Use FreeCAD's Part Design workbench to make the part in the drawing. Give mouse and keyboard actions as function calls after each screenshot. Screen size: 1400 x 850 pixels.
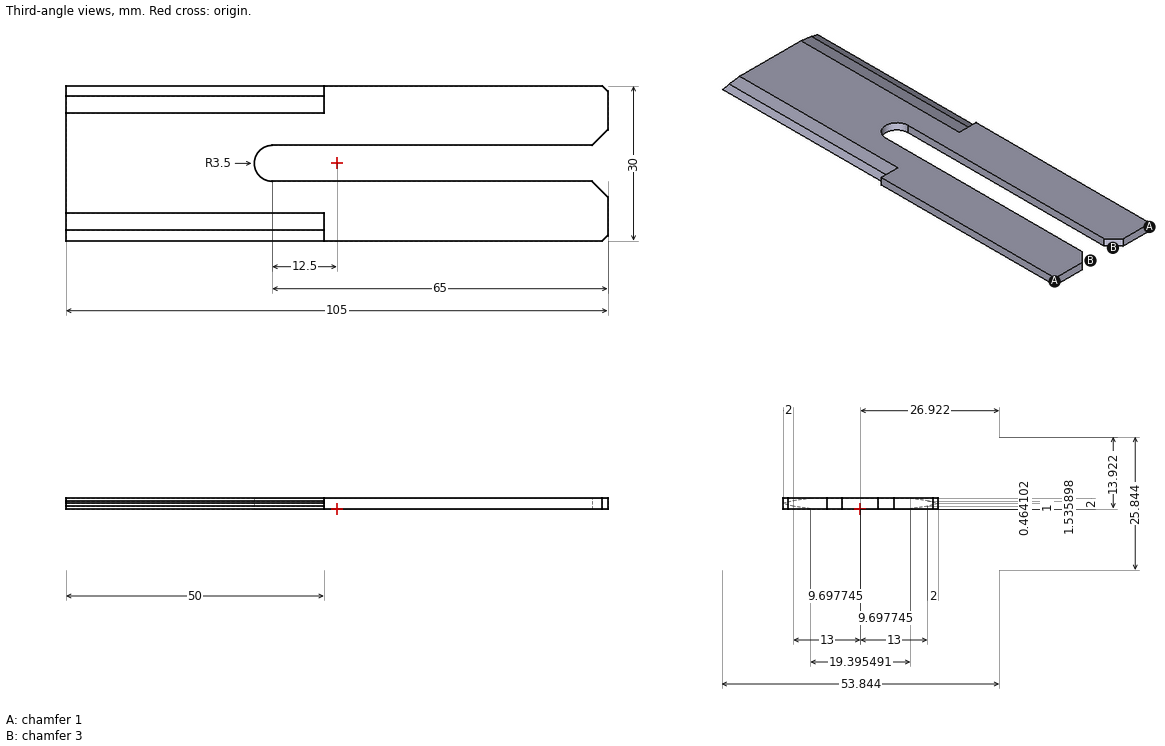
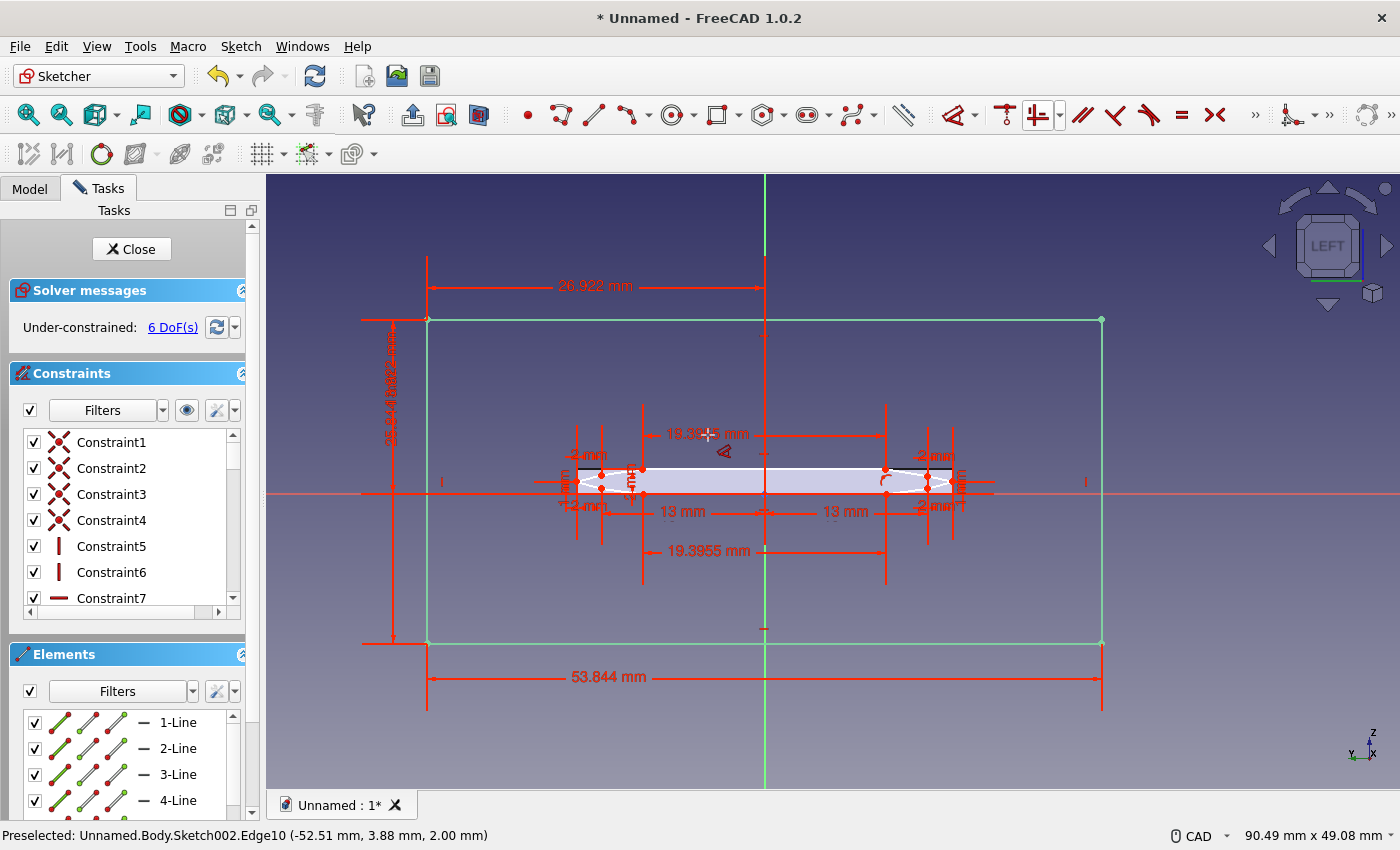
click(886, 494)
click(825, 552)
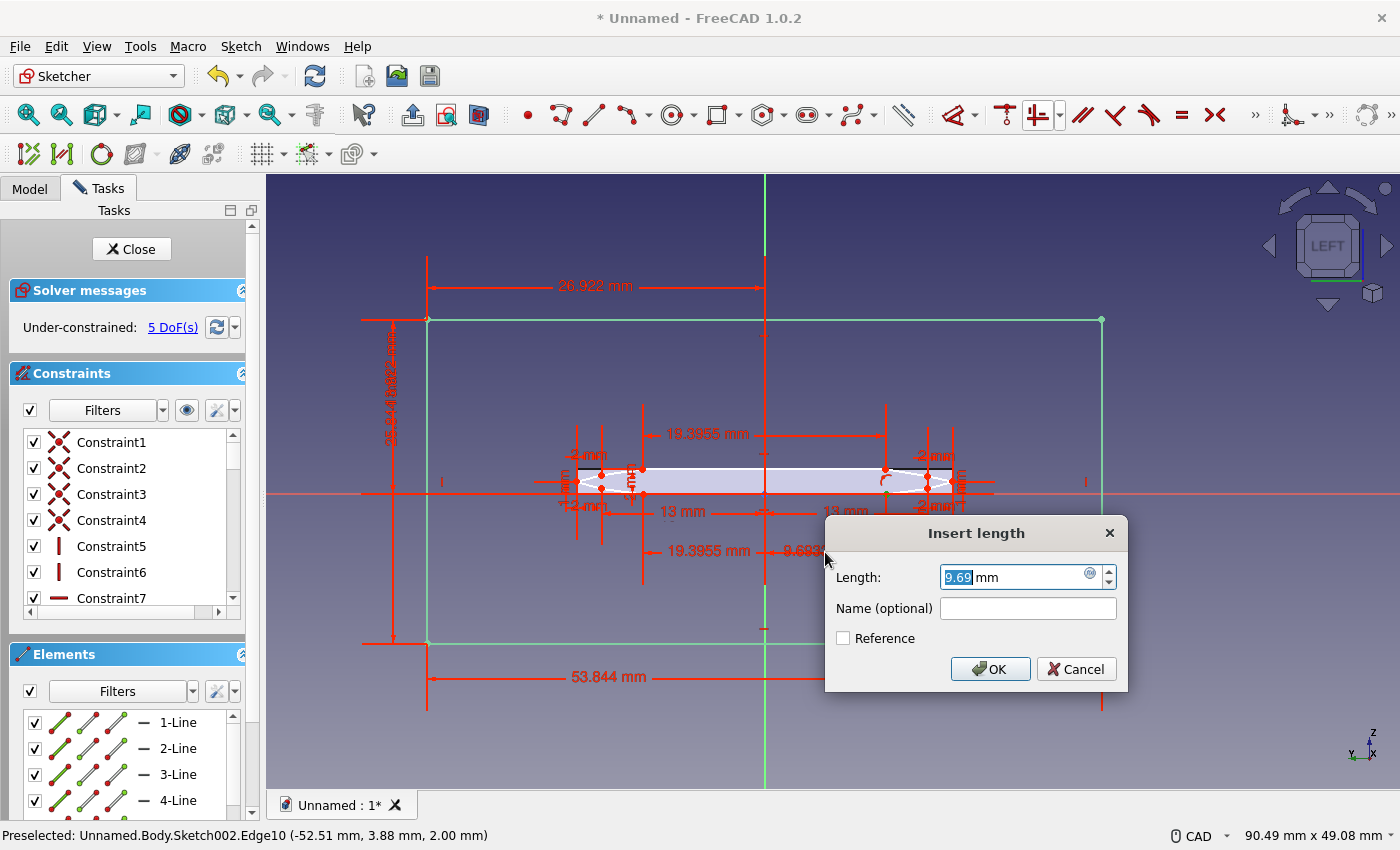
text(9.697745)
key(Return)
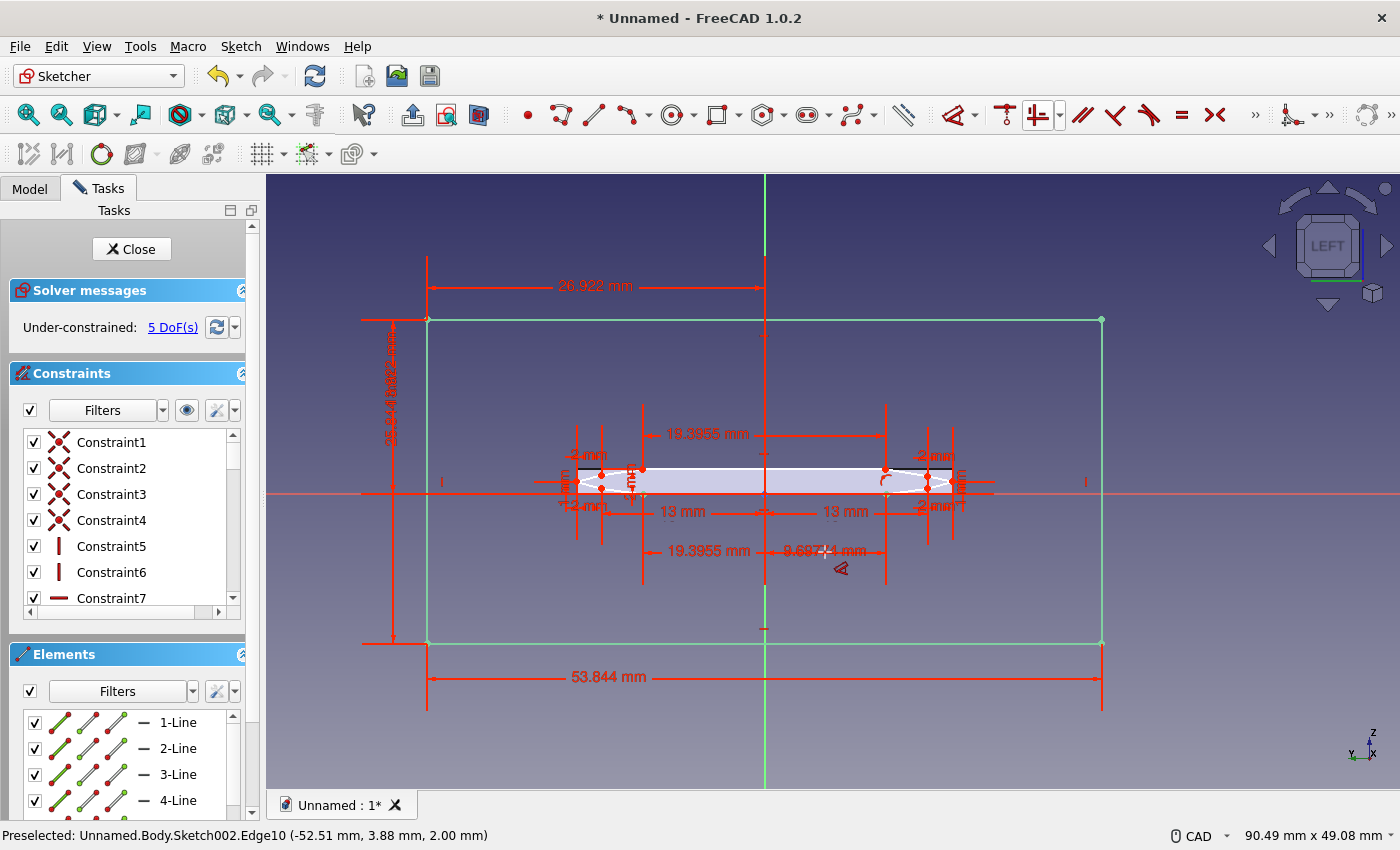
scroll(602, 489, up, 10)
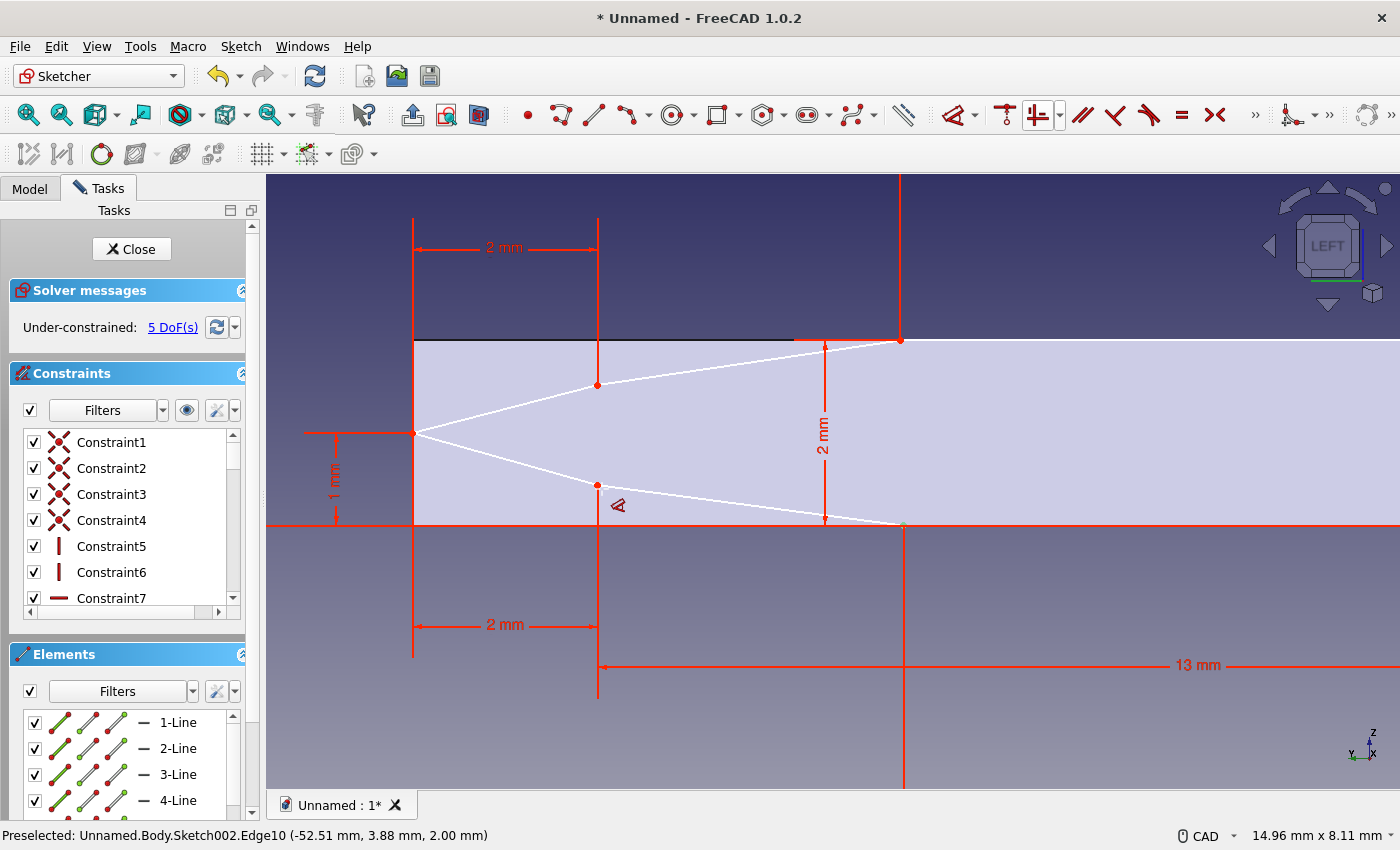
click(598, 485)
click(564, 505)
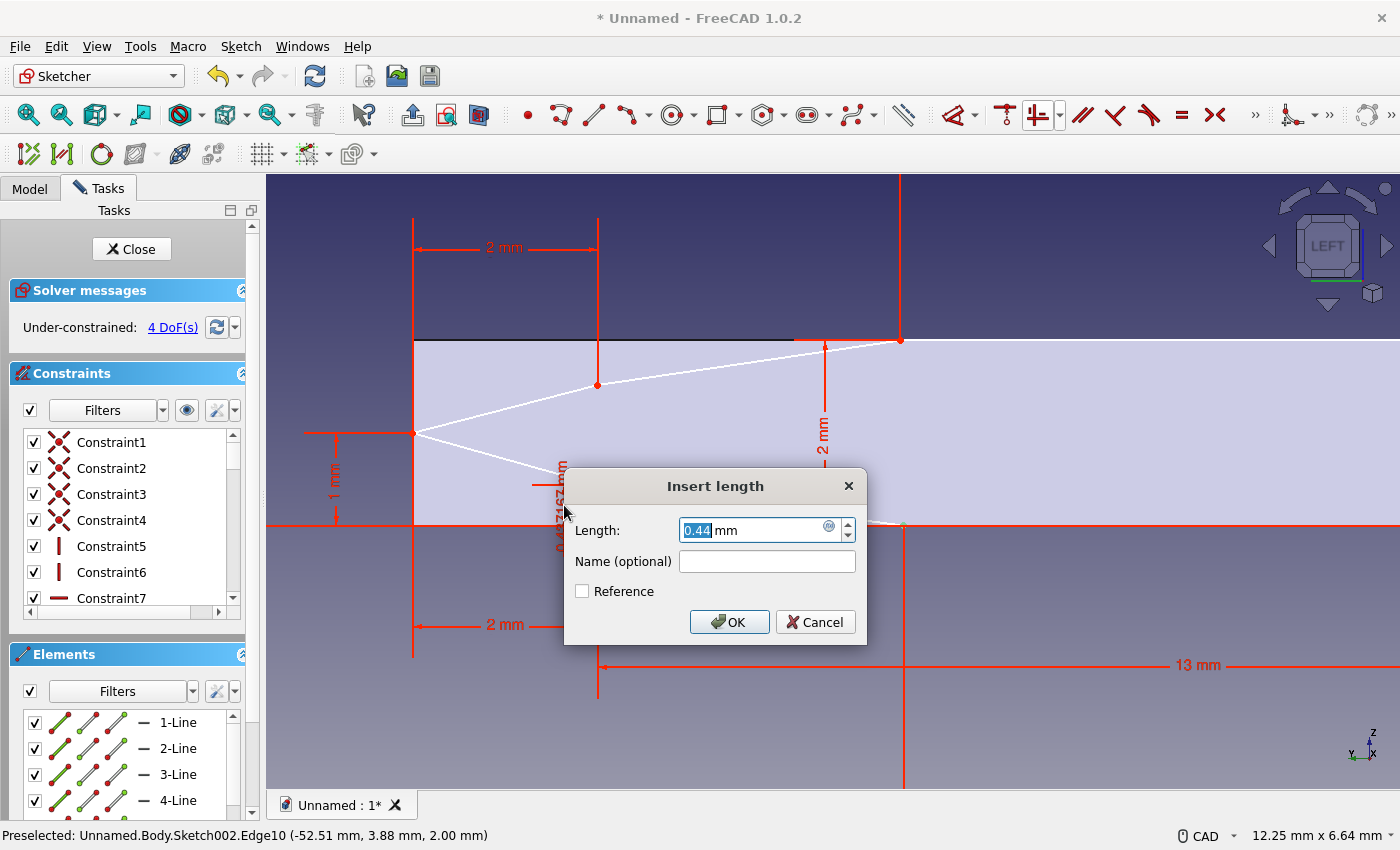
text(0.464102)
key(Return)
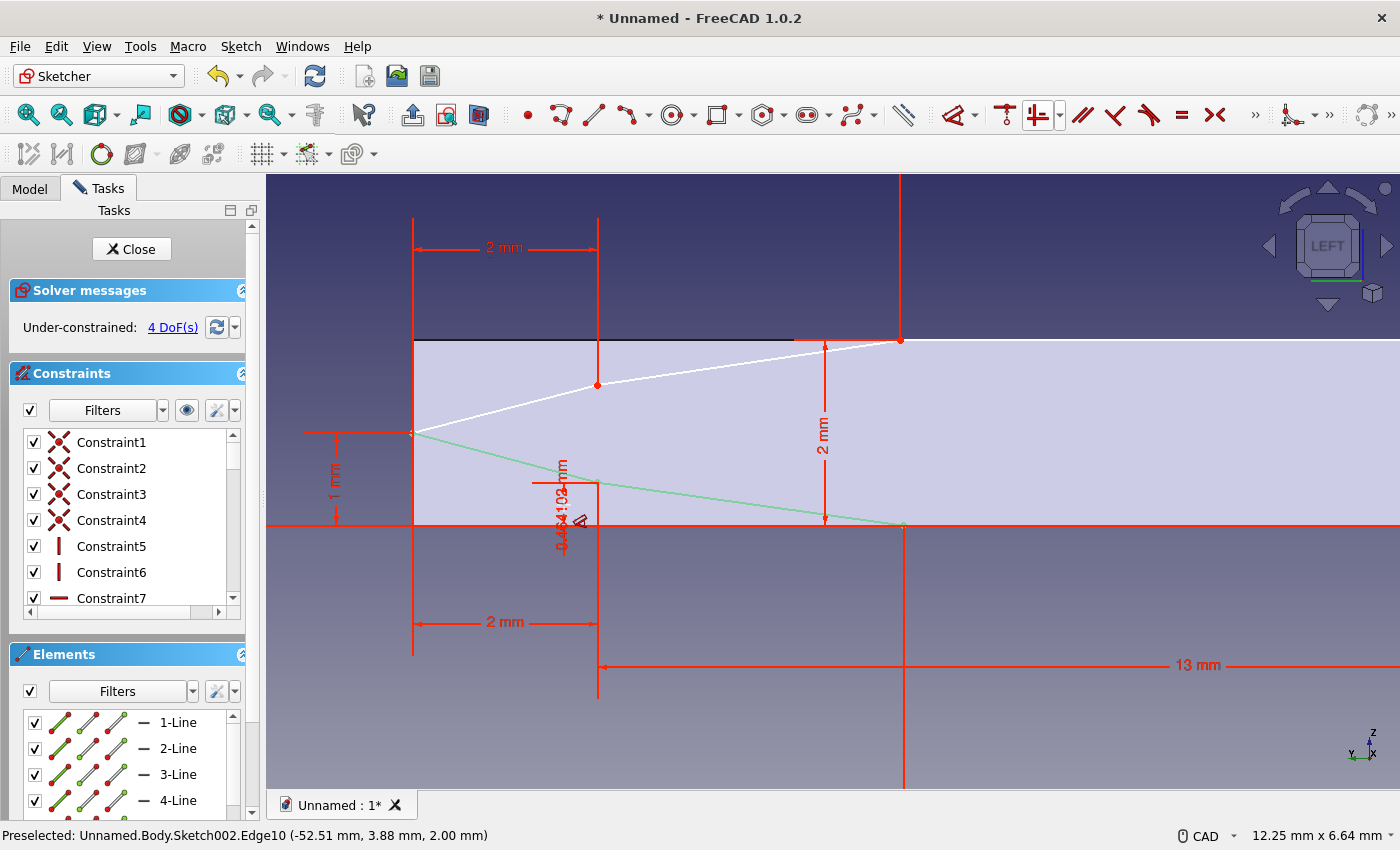
scroll(602, 489, down, 10)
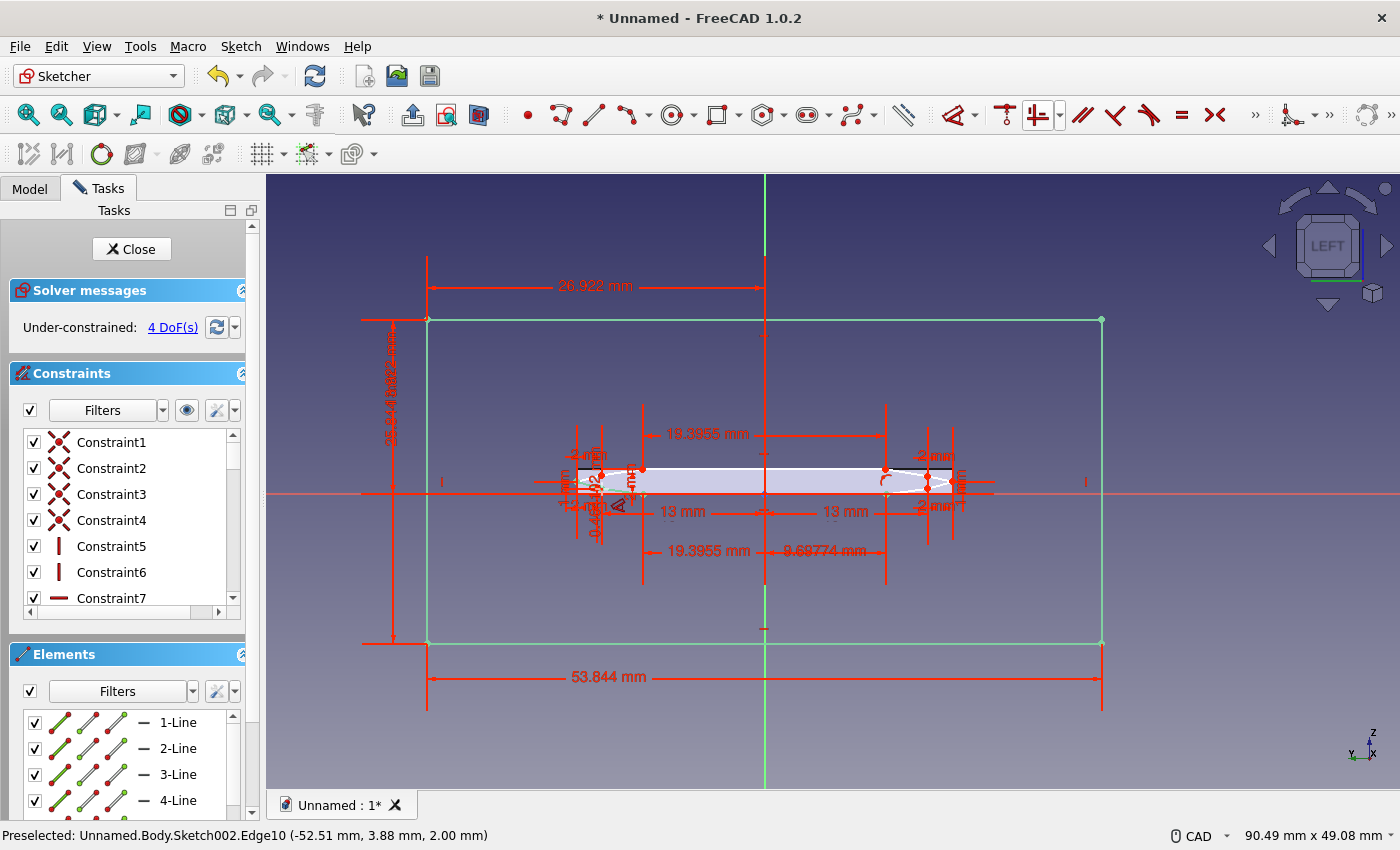
scroll(602, 475, up, 4)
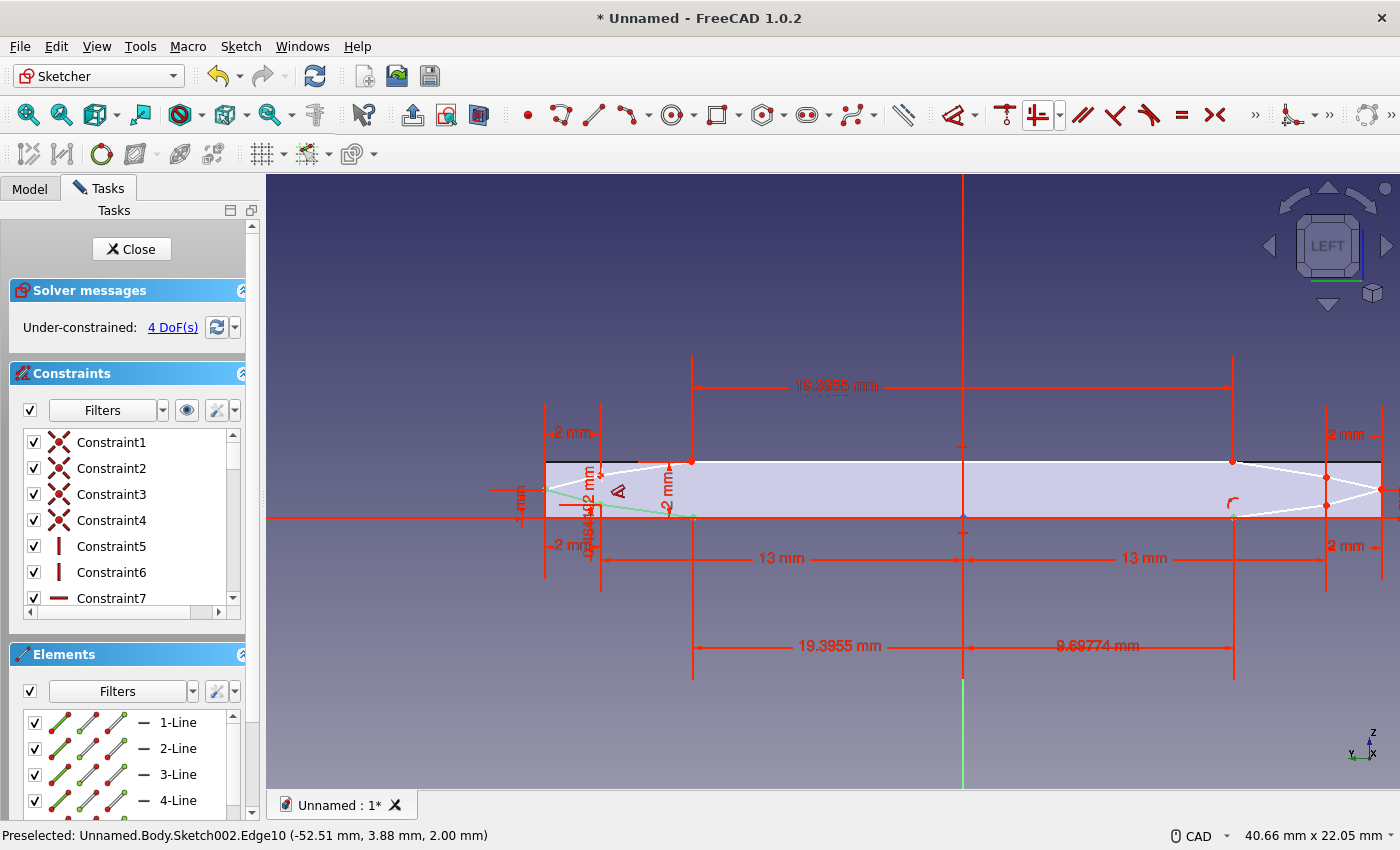
click(601, 475)
click(997, 496)